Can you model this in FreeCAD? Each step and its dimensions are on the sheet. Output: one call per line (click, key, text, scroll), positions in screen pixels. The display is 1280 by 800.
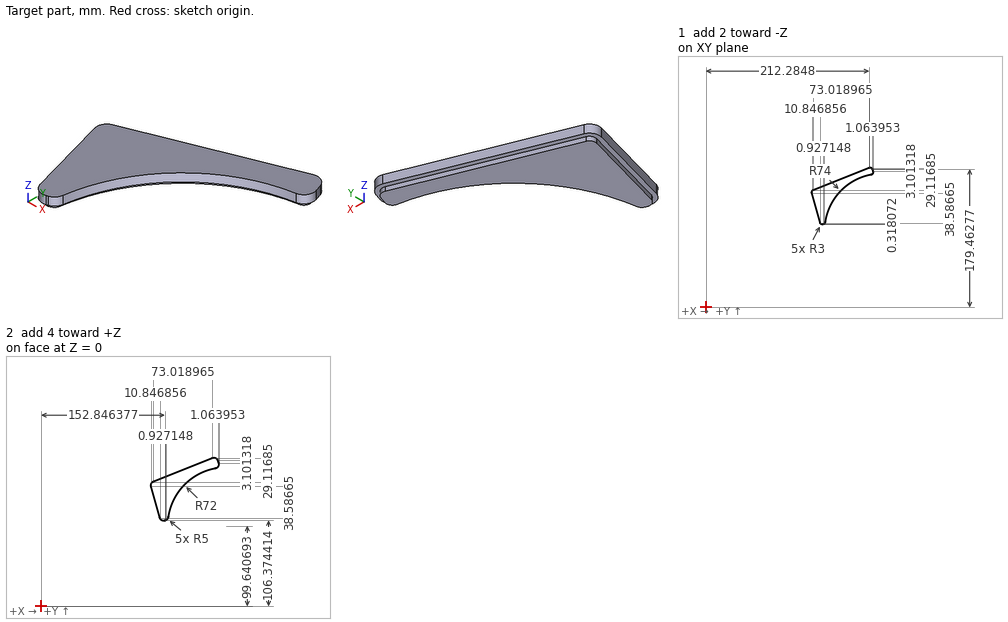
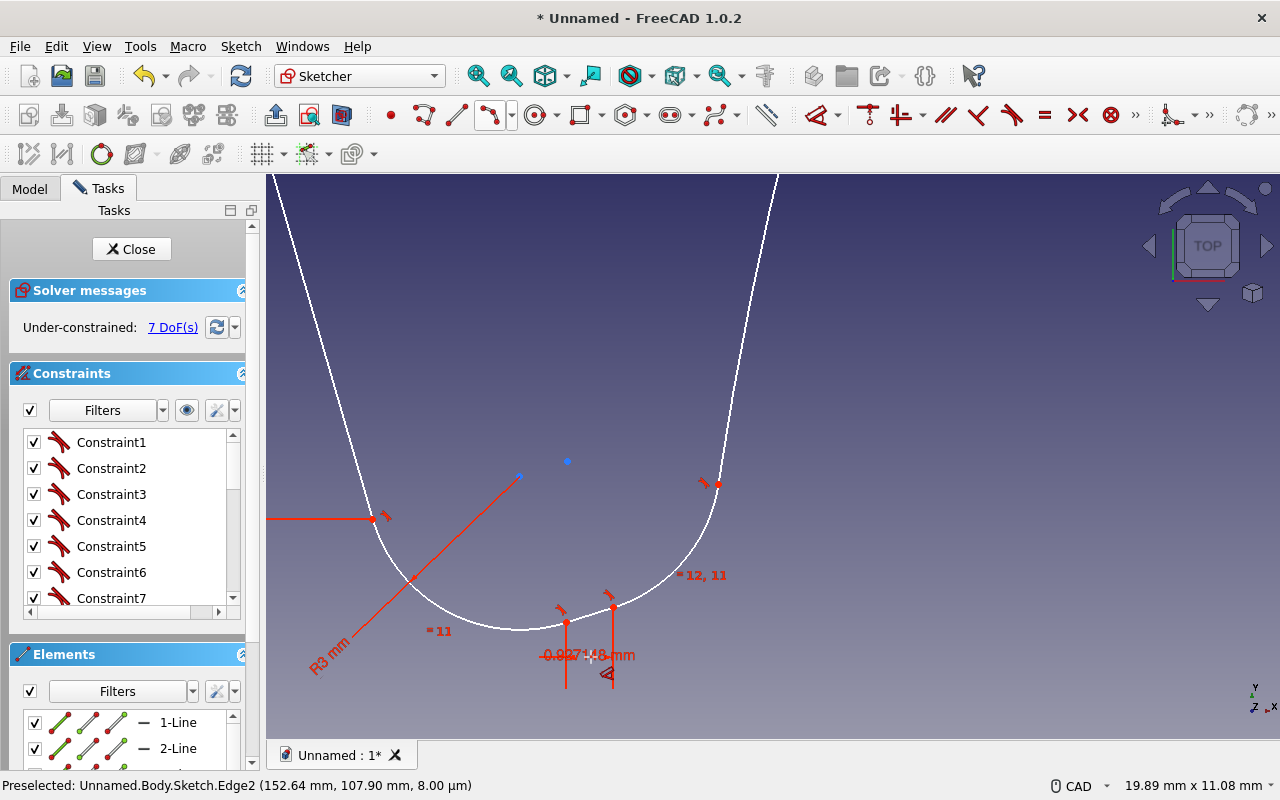
scroll(580, 618, up, 5)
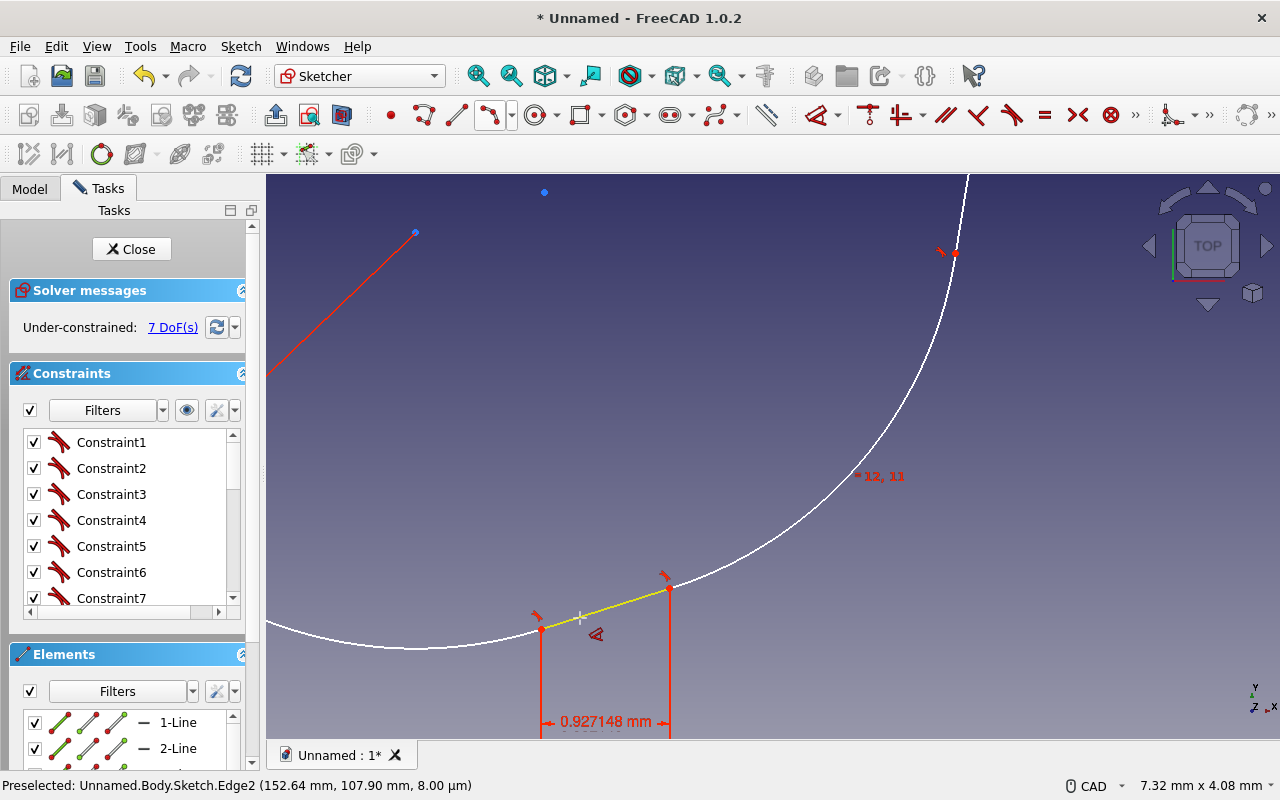
click(580, 617)
click(507, 609)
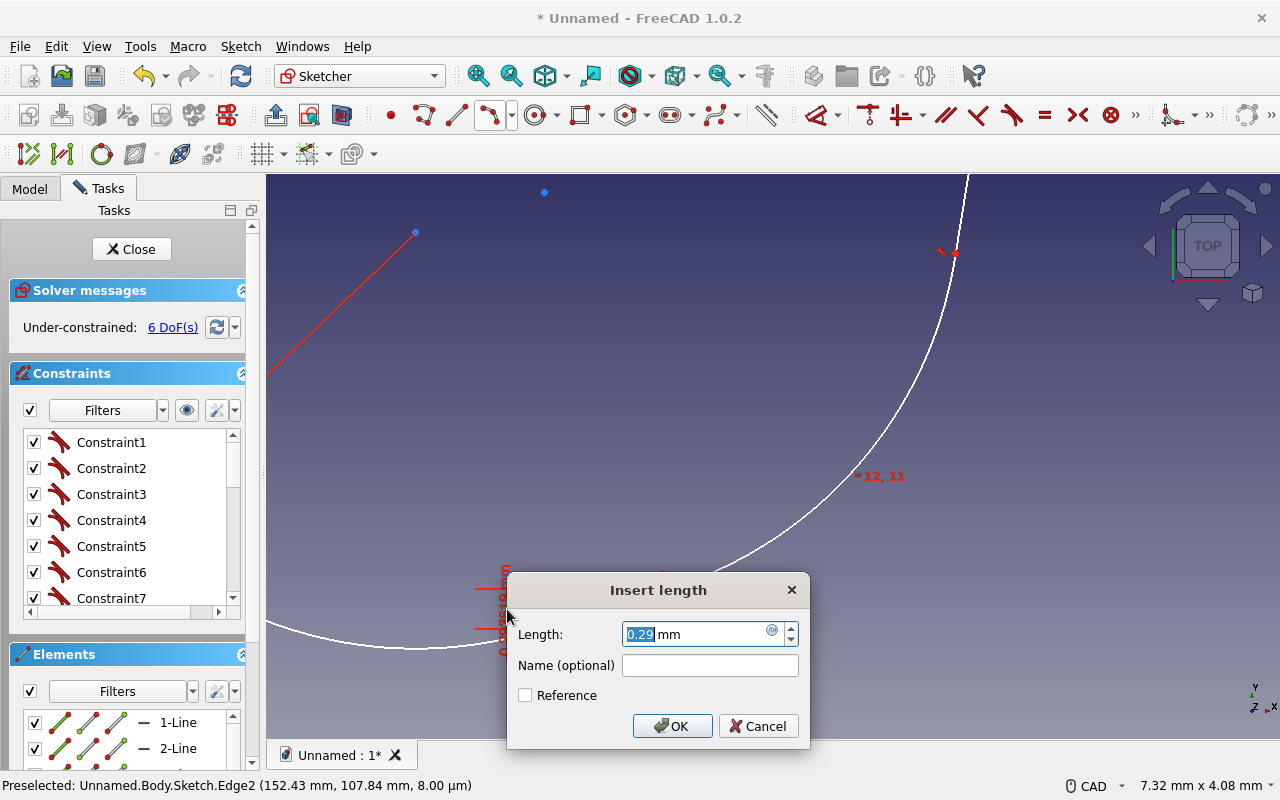
text(0.318072)
key(Return)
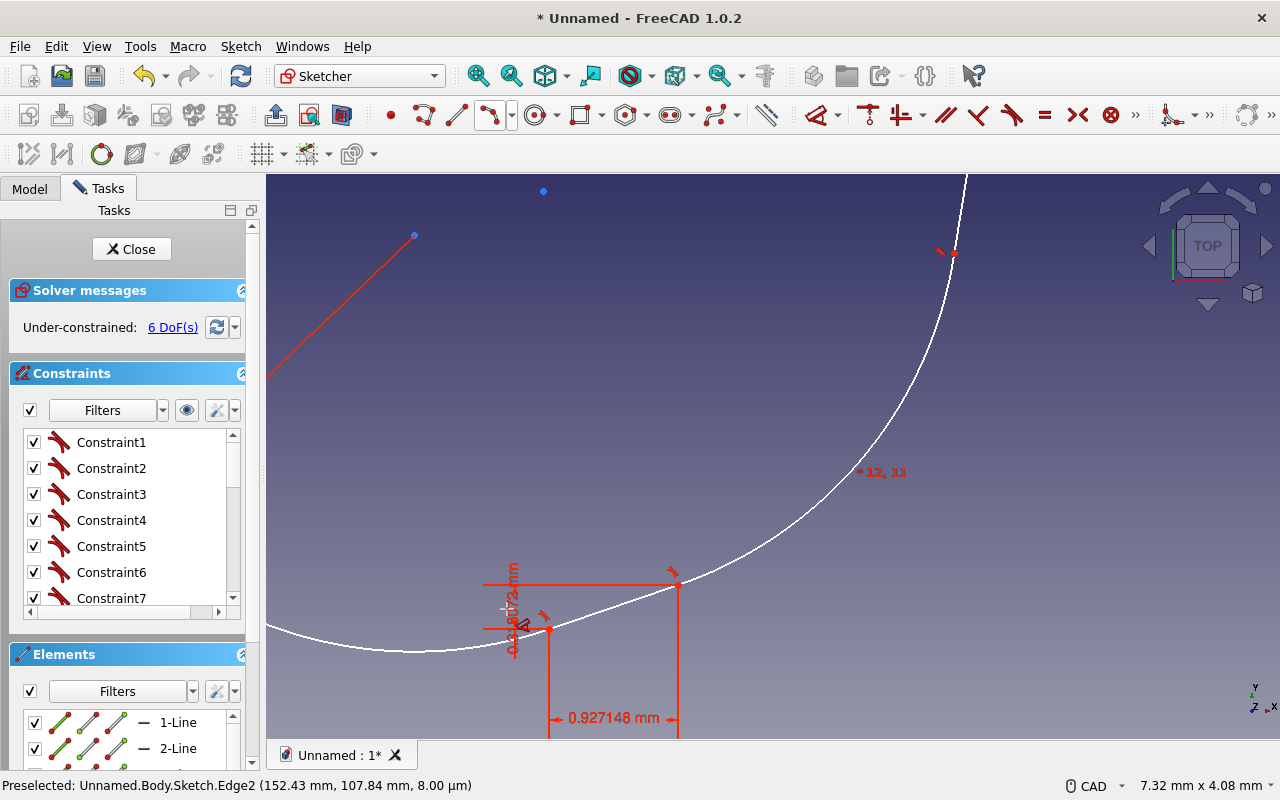
scroll(563, 666, down, 16)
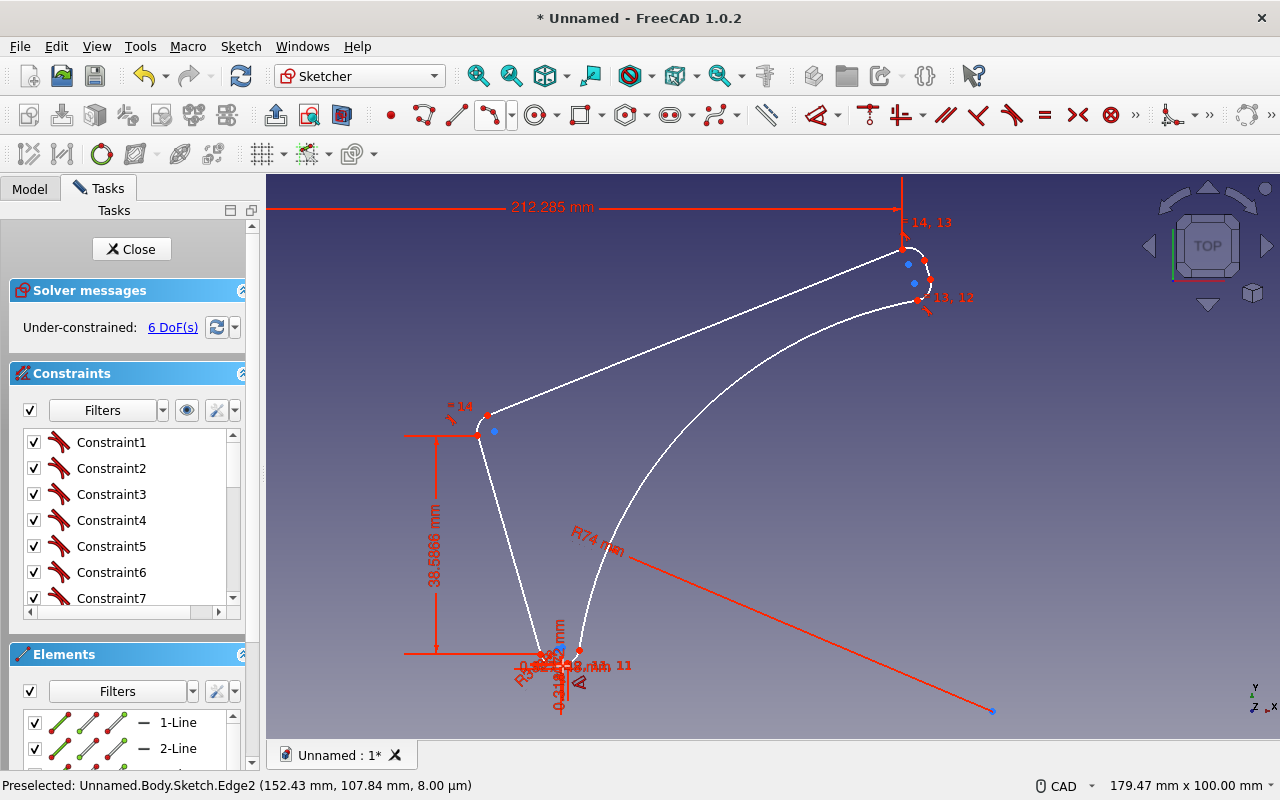
scroll(929, 273, up, 10)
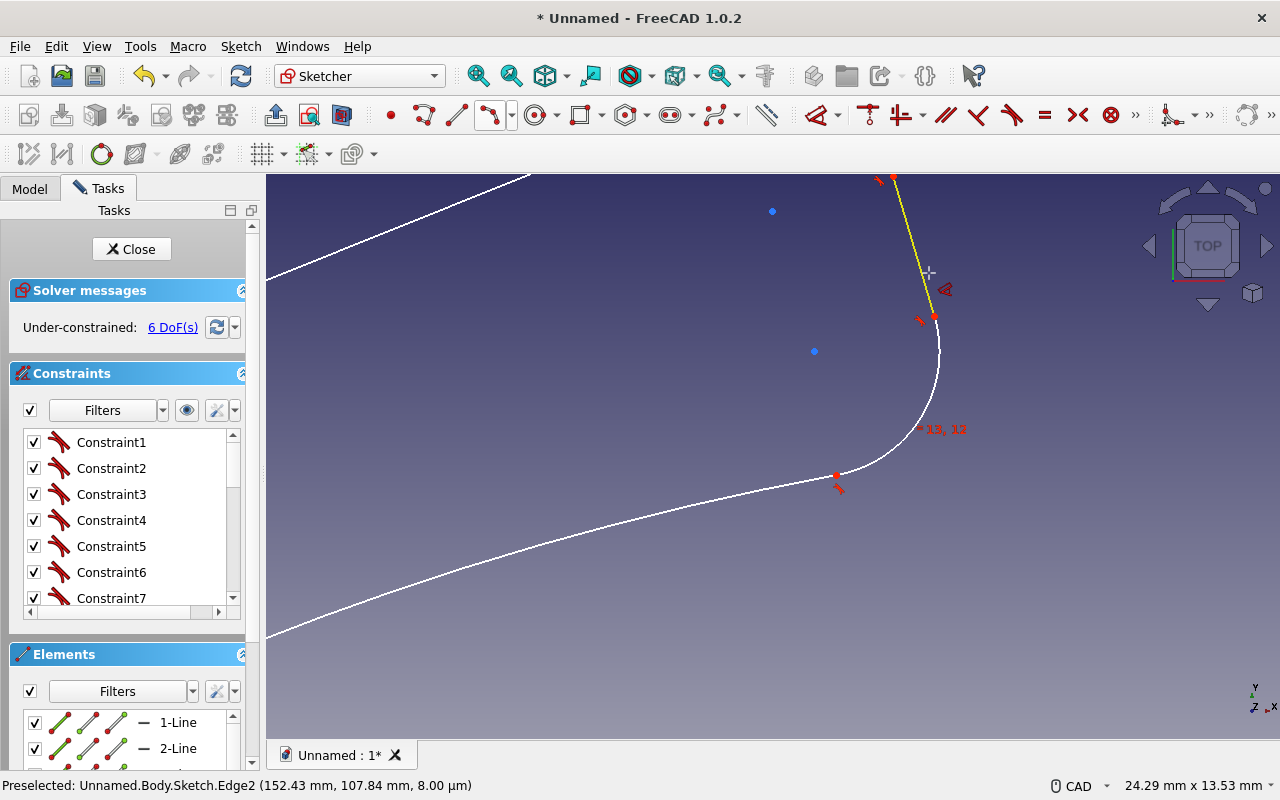
click(922, 274)
click(914, 350)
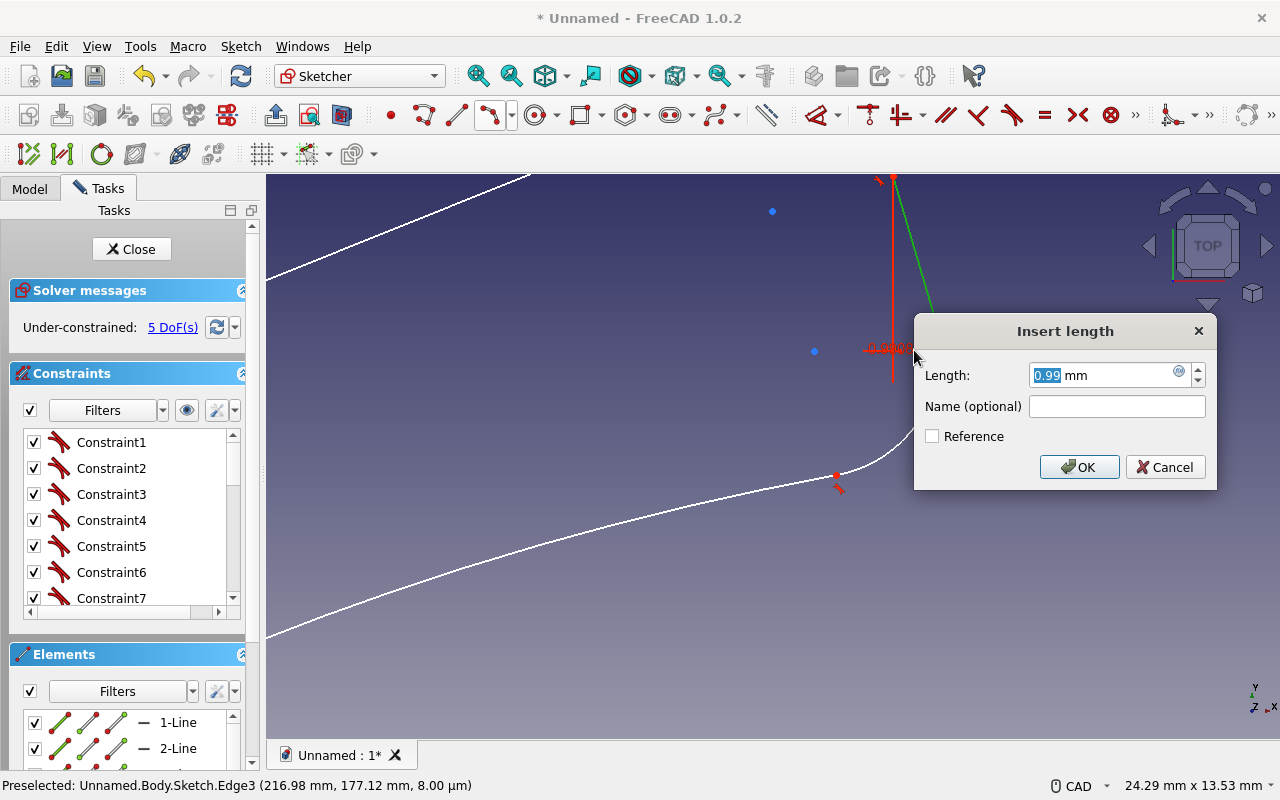
text(1.063953)
key(Return)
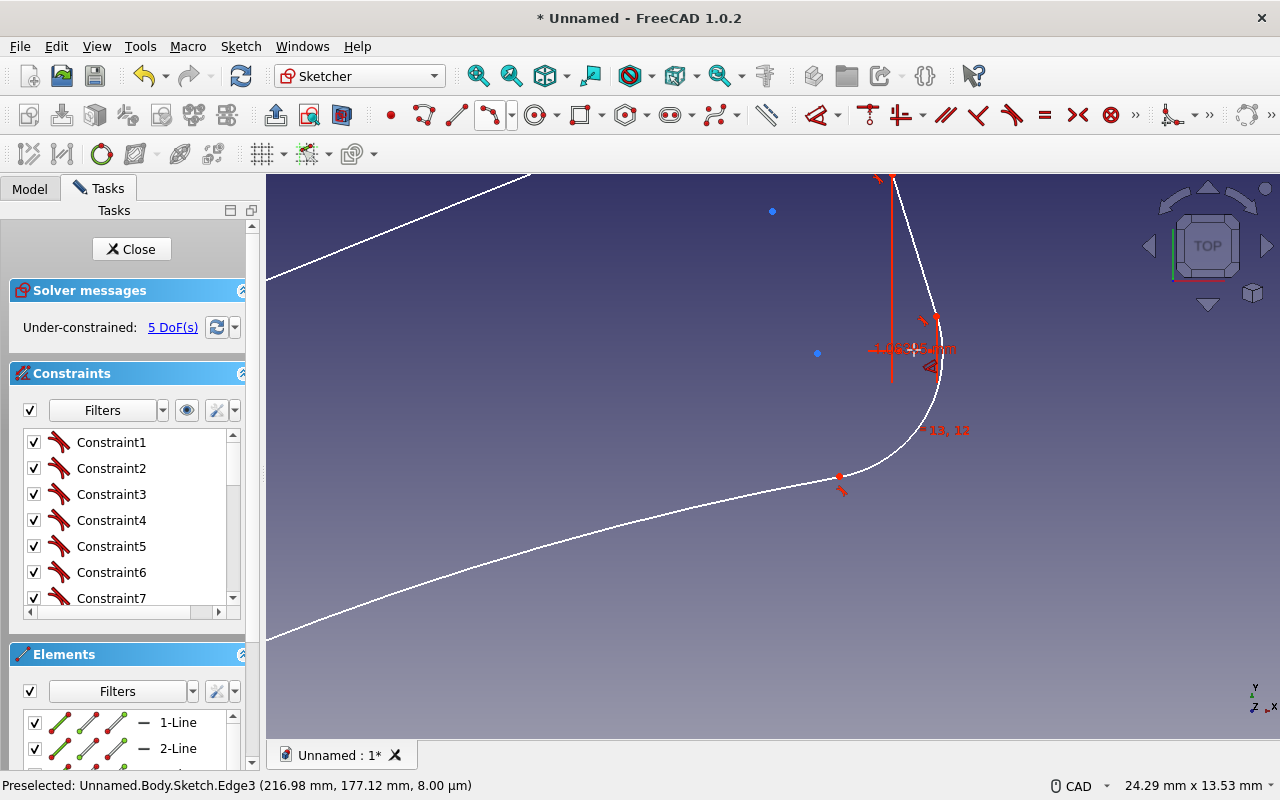
scroll(883, 310, down, 11)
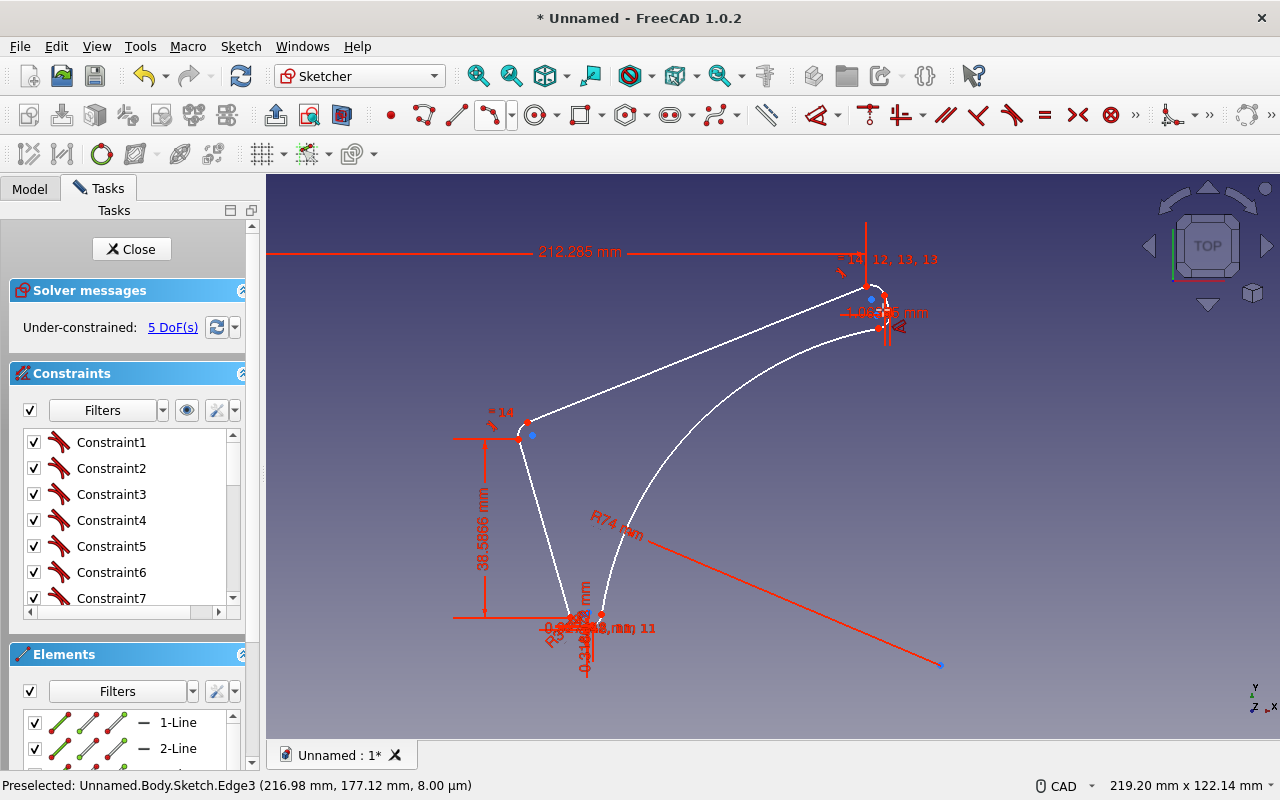
scroll(888, 306, up, 6)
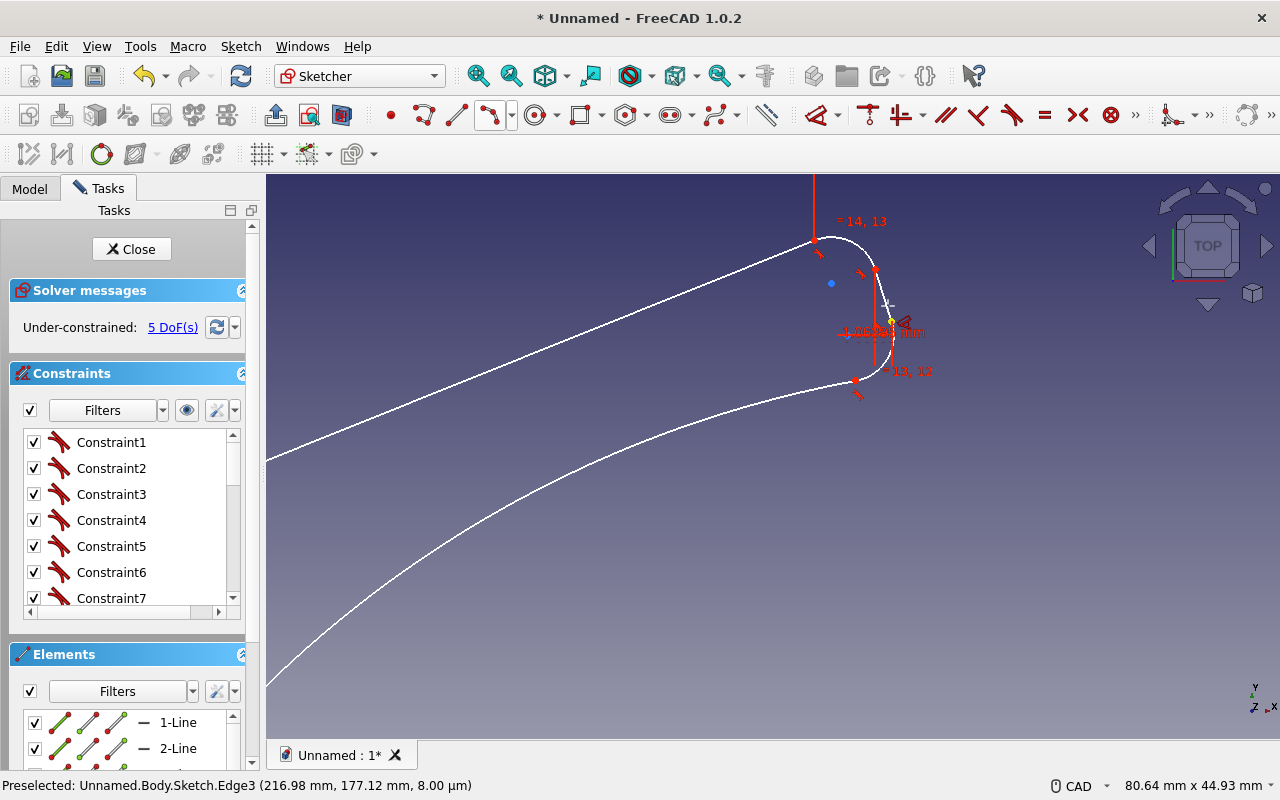
click(887, 306)
click(926, 296)